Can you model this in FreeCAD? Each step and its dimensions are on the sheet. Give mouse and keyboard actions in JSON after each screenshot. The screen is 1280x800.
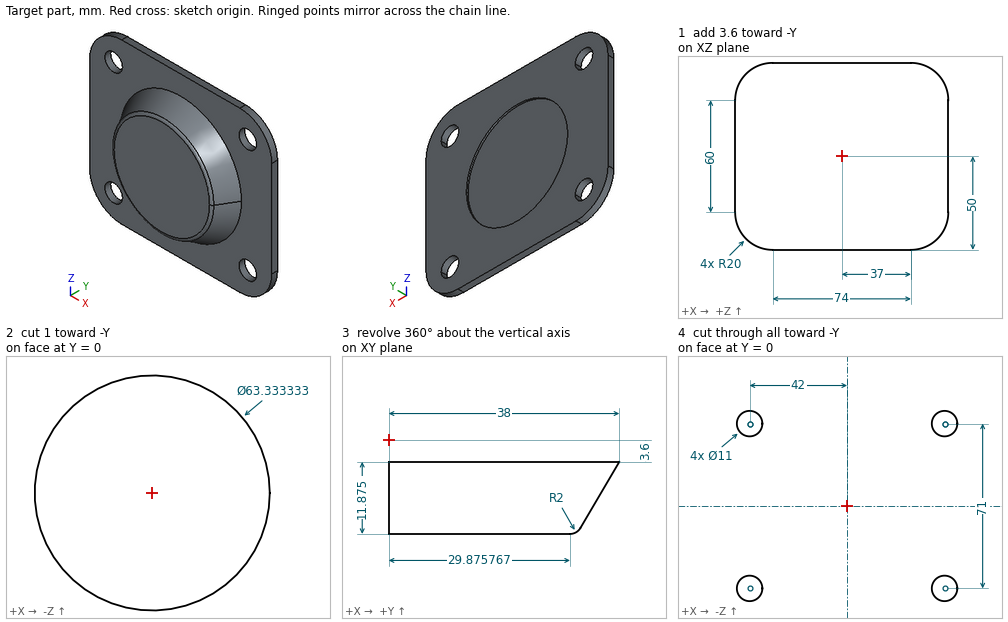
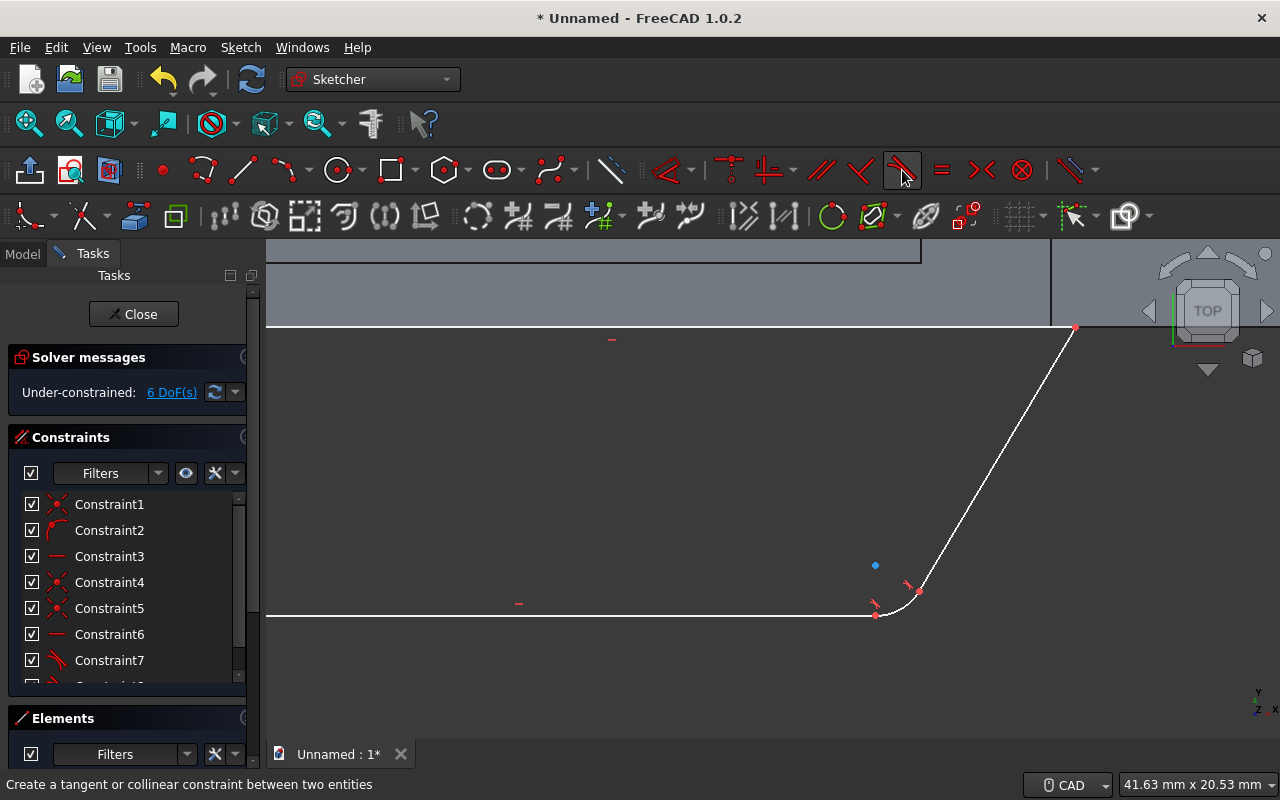
{"action": "scroll", "coordinate": [892, 614], "scroll_direction": "down", "scroll_amount": 2}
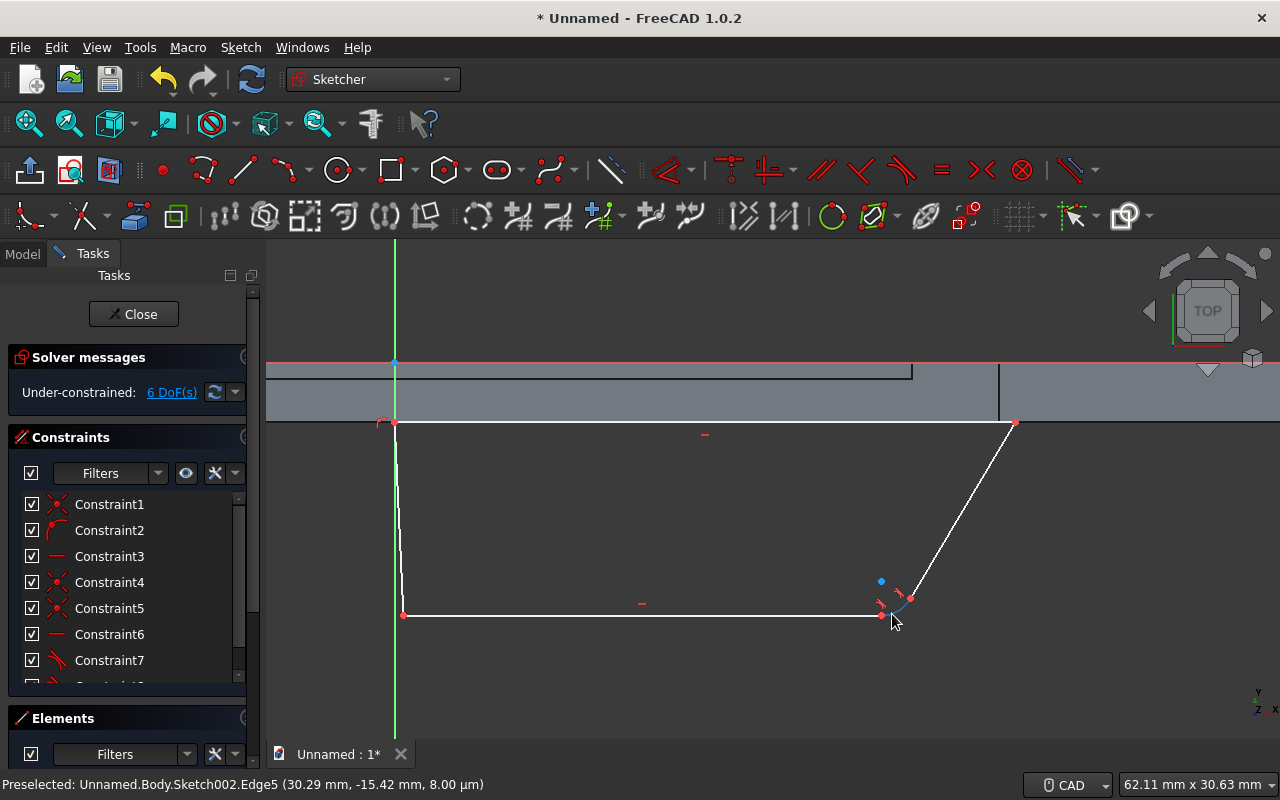
{"action": "left_click", "coordinate": [397, 480]}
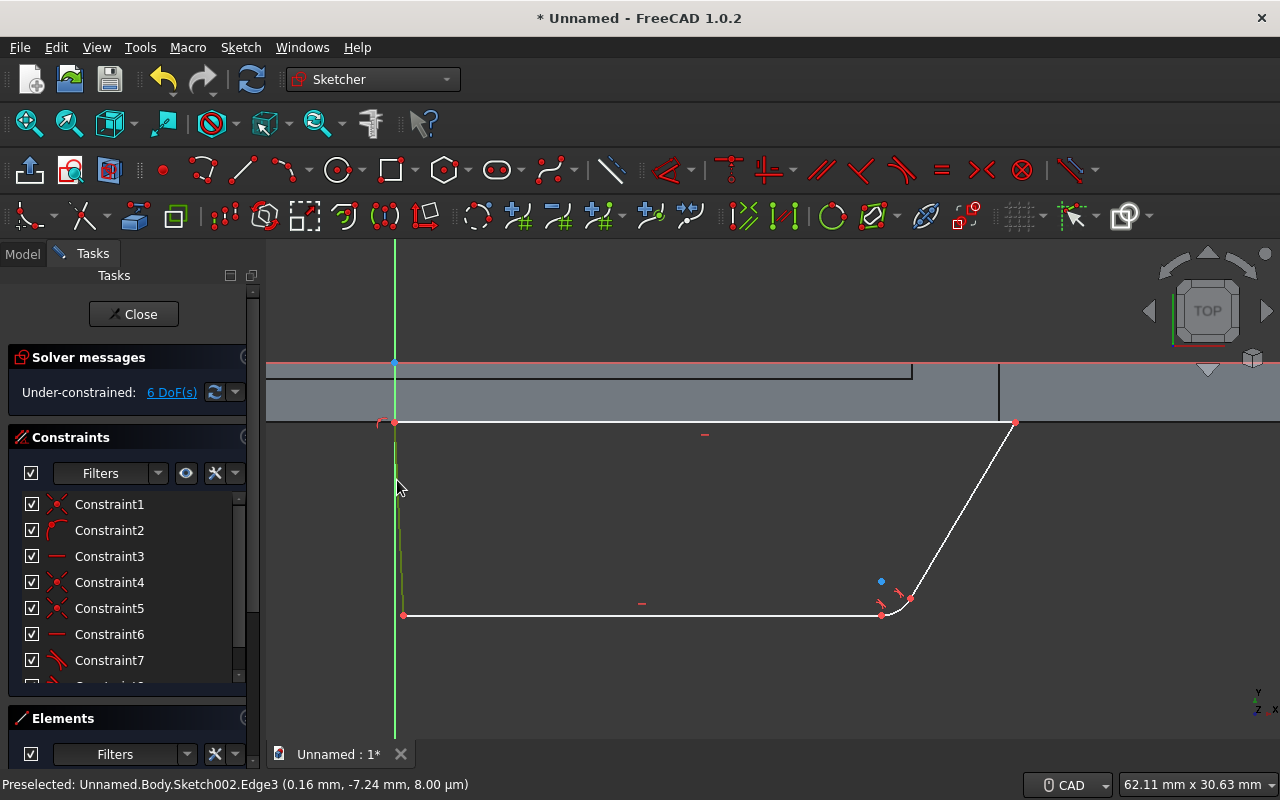
{"action": "left_click", "coordinate": [796, 170]}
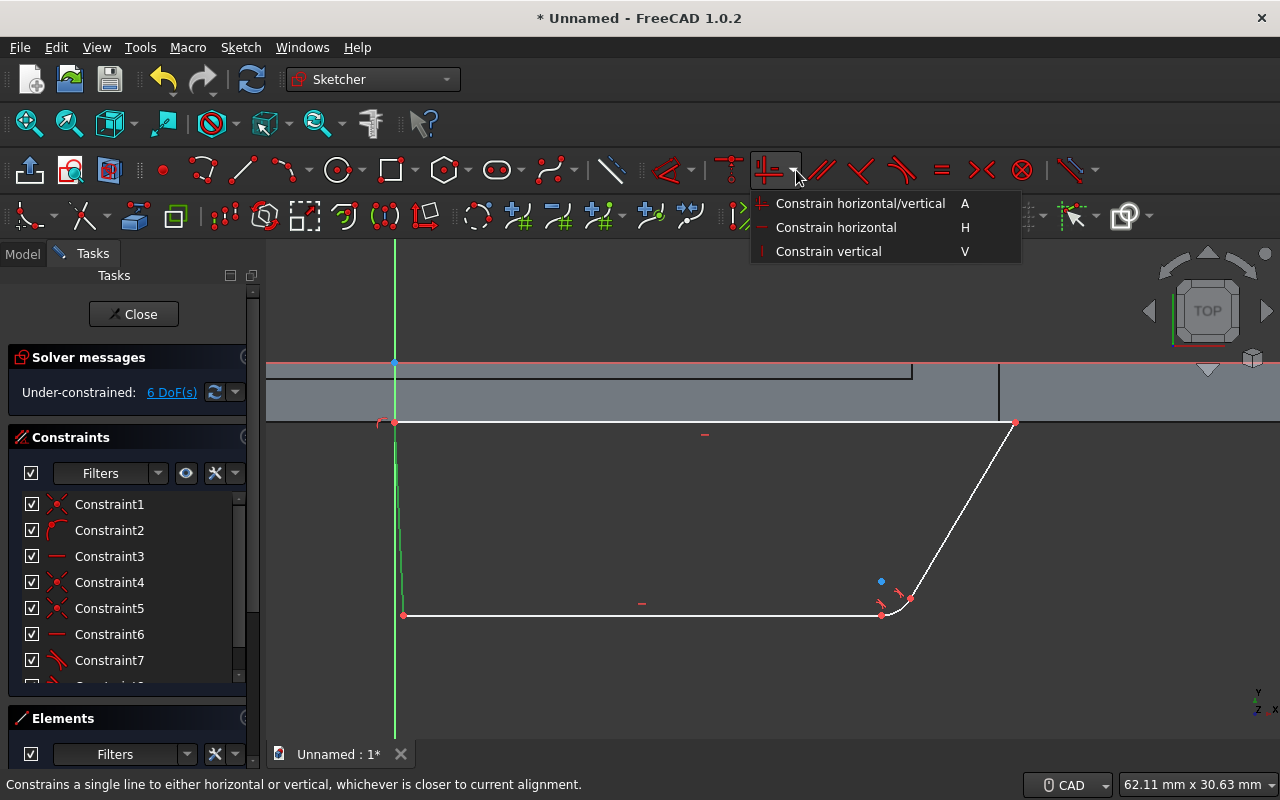
{"action": "left_click", "coordinate": [886, 251]}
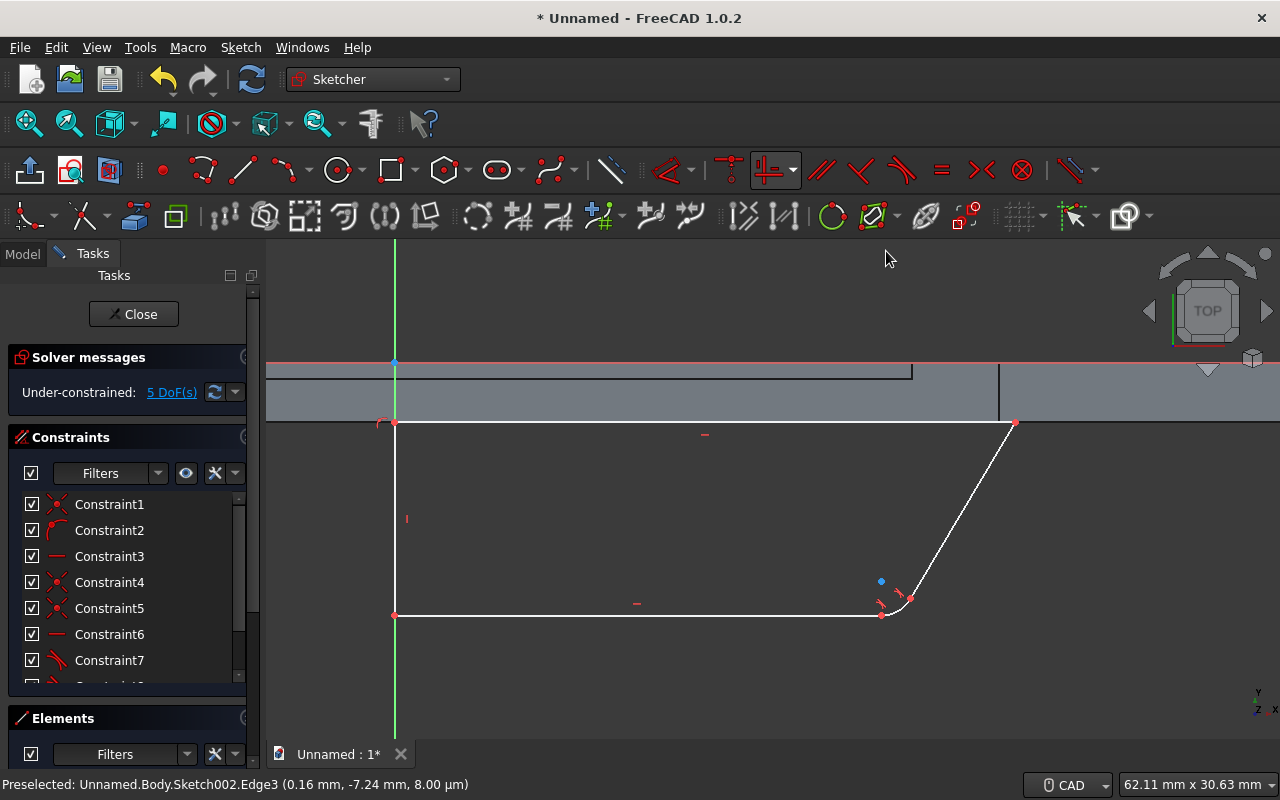
{"action": "left_click", "coordinate": [666, 170]}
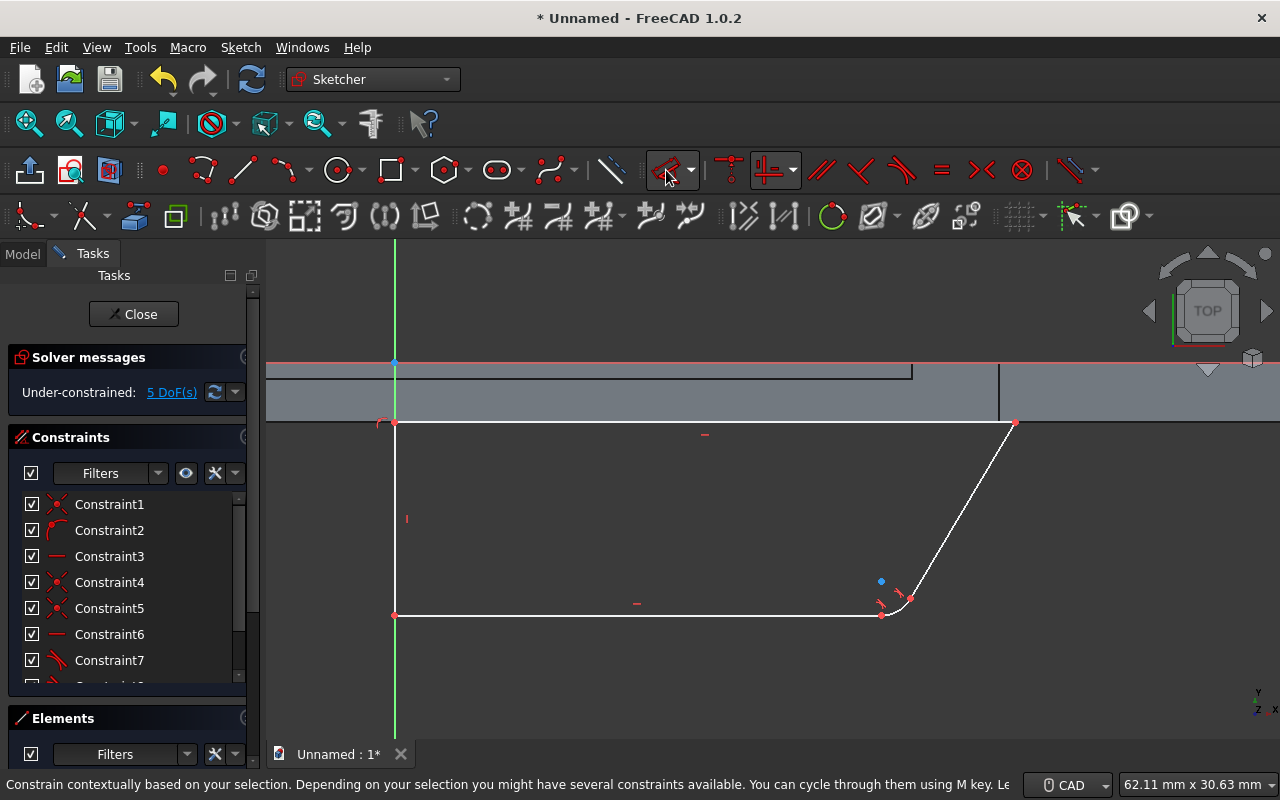
{"action": "scroll", "coordinate": [892, 614], "scroll_direction": "up", "scroll_amount": 2}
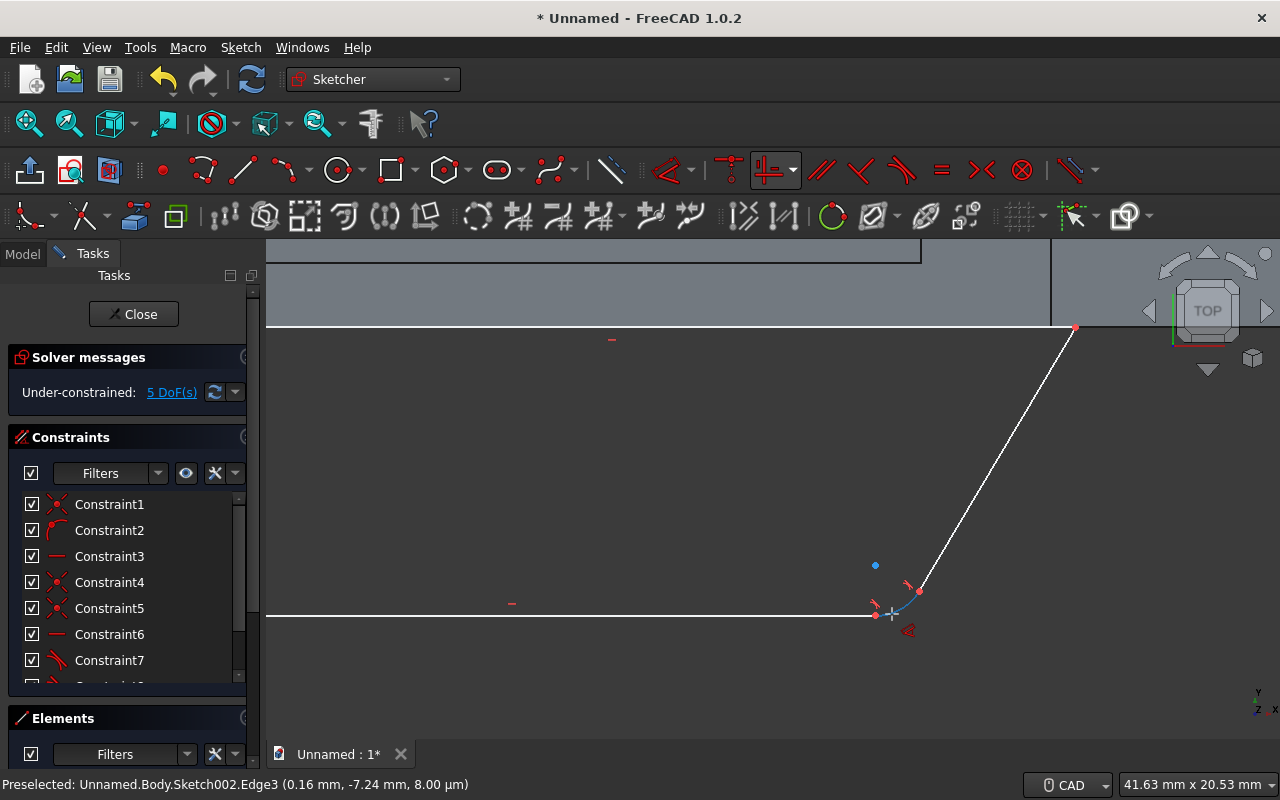
{"action": "left_click", "coordinate": [891, 614]}
{"action": "left_click", "coordinate": [901, 645]}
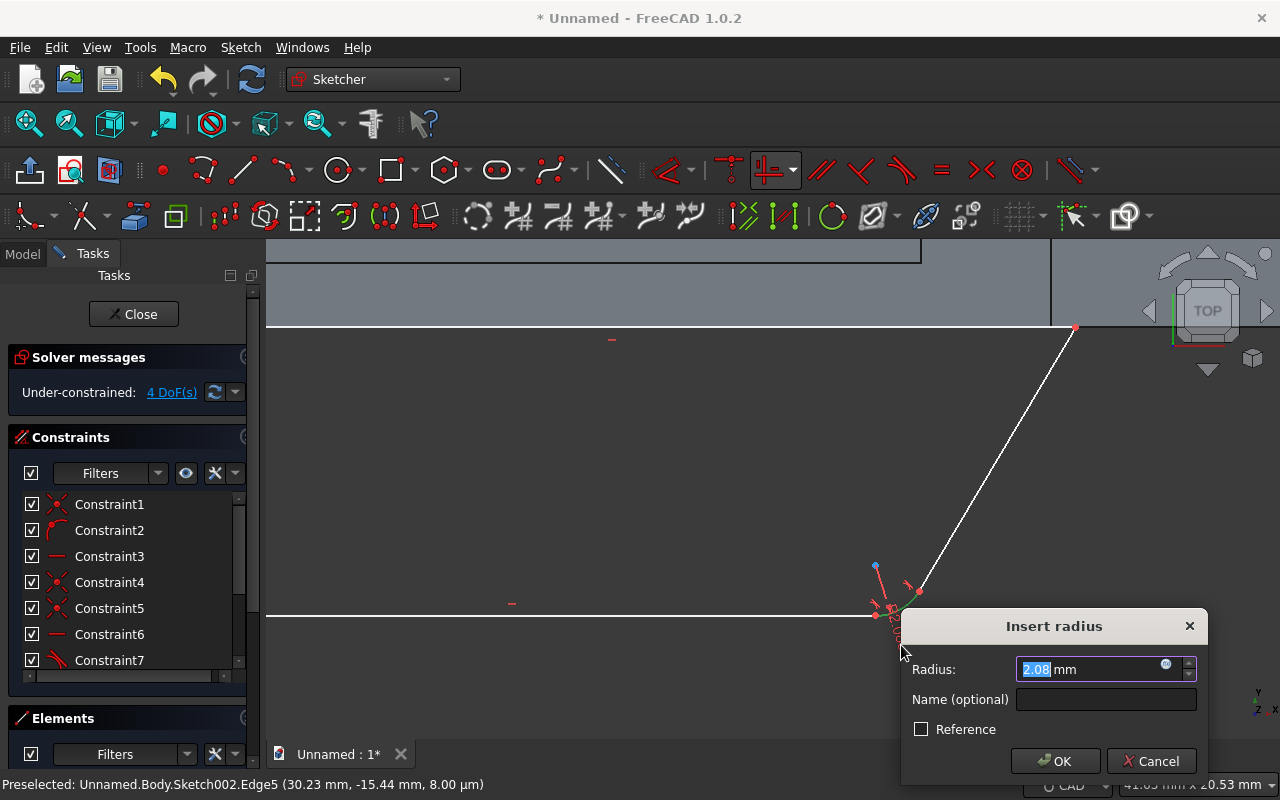
{"action": "type", "text": "2"}
{"action": "key", "text": "Return"}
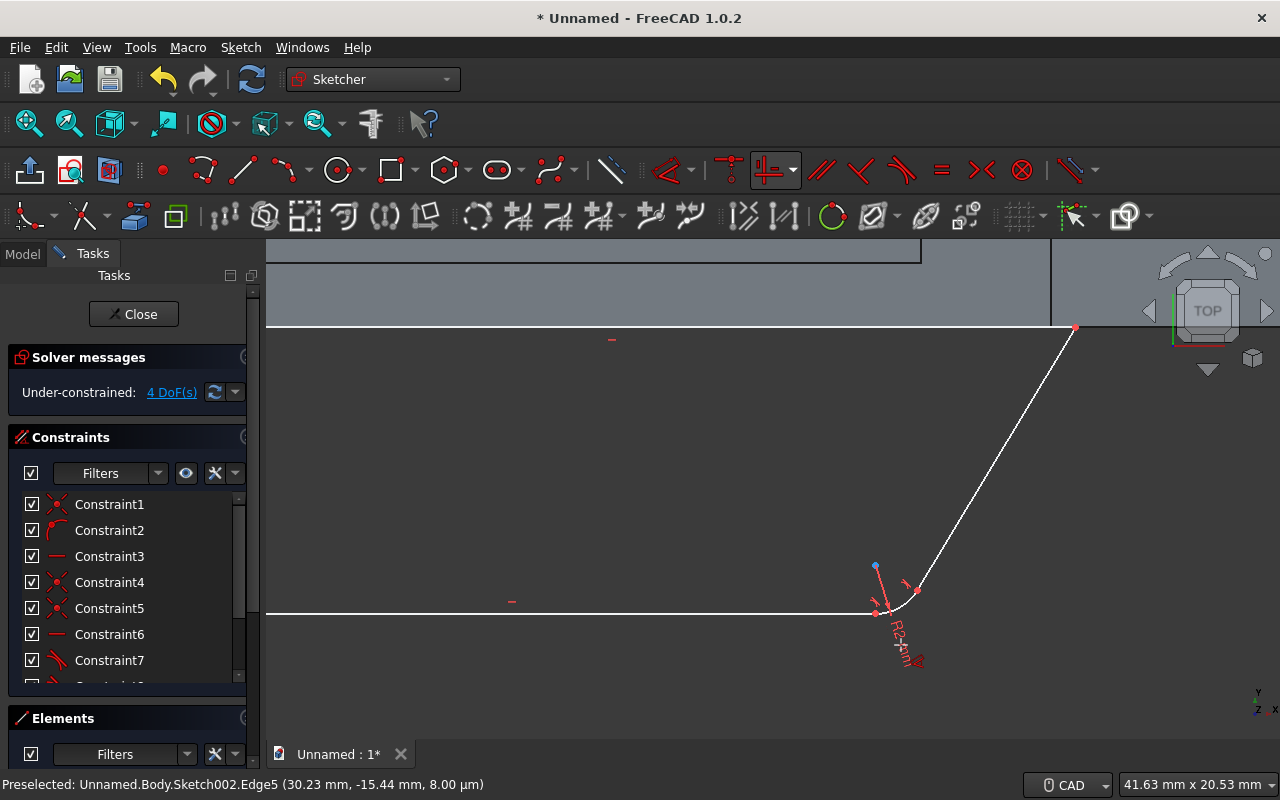
{"action": "left_click", "coordinate": [798, 327]}
{"action": "left_click", "coordinate": [685, 293]}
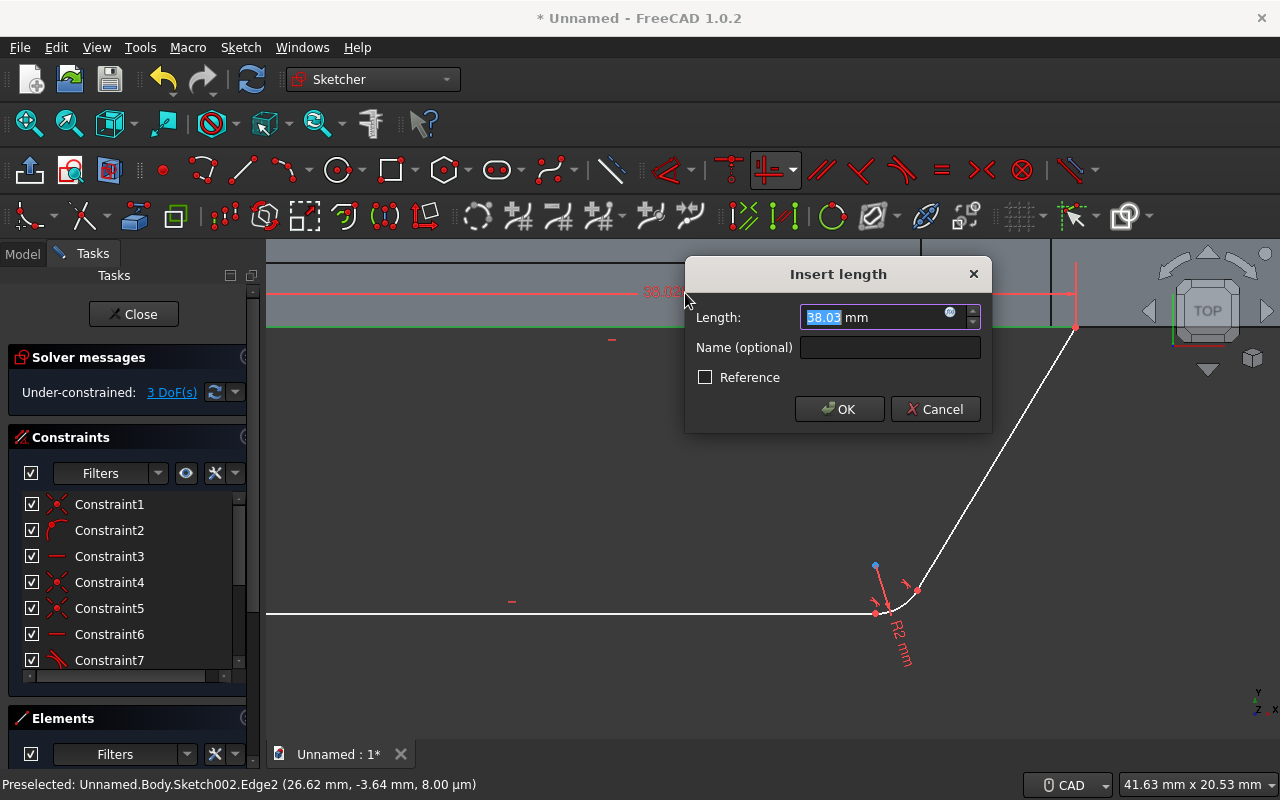
{"action": "type", "text": "38"}
{"action": "key", "text": "Return"}